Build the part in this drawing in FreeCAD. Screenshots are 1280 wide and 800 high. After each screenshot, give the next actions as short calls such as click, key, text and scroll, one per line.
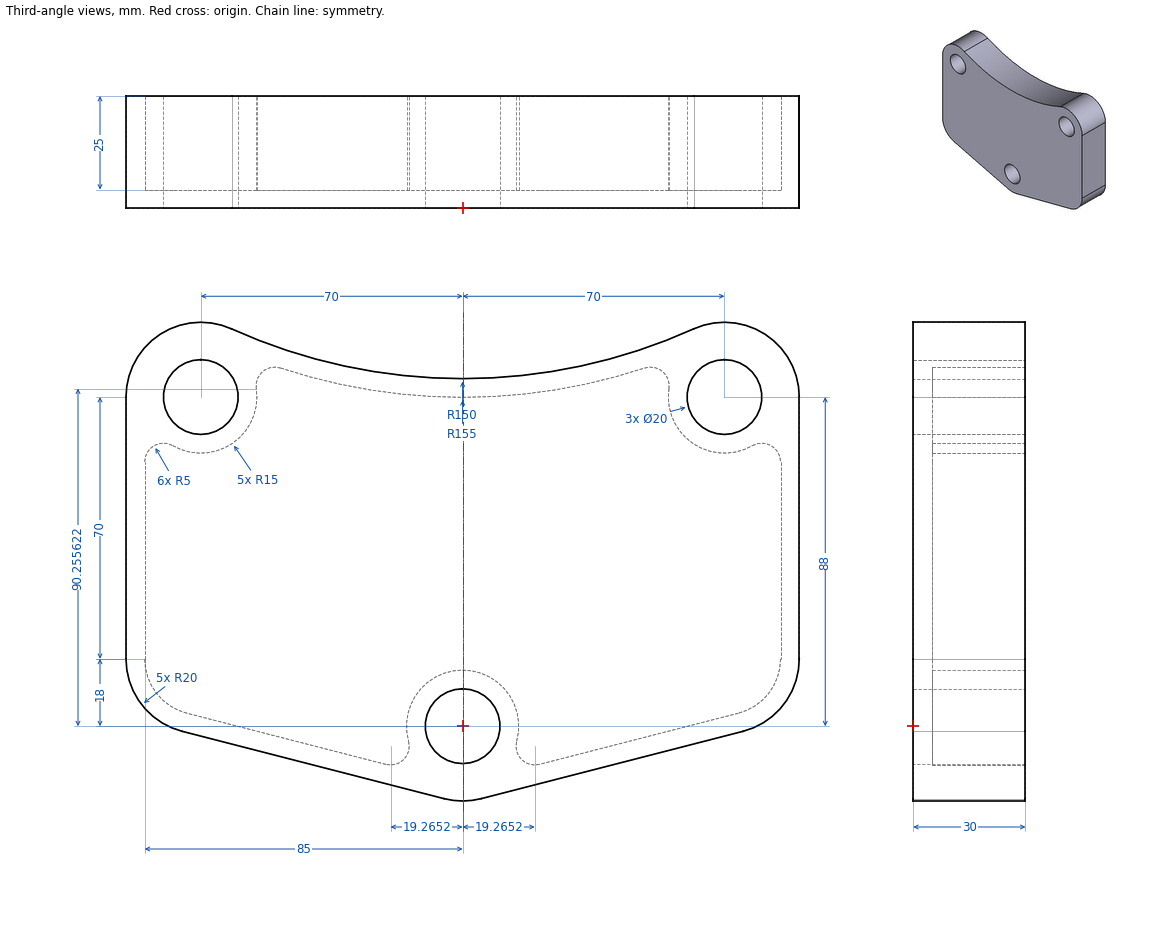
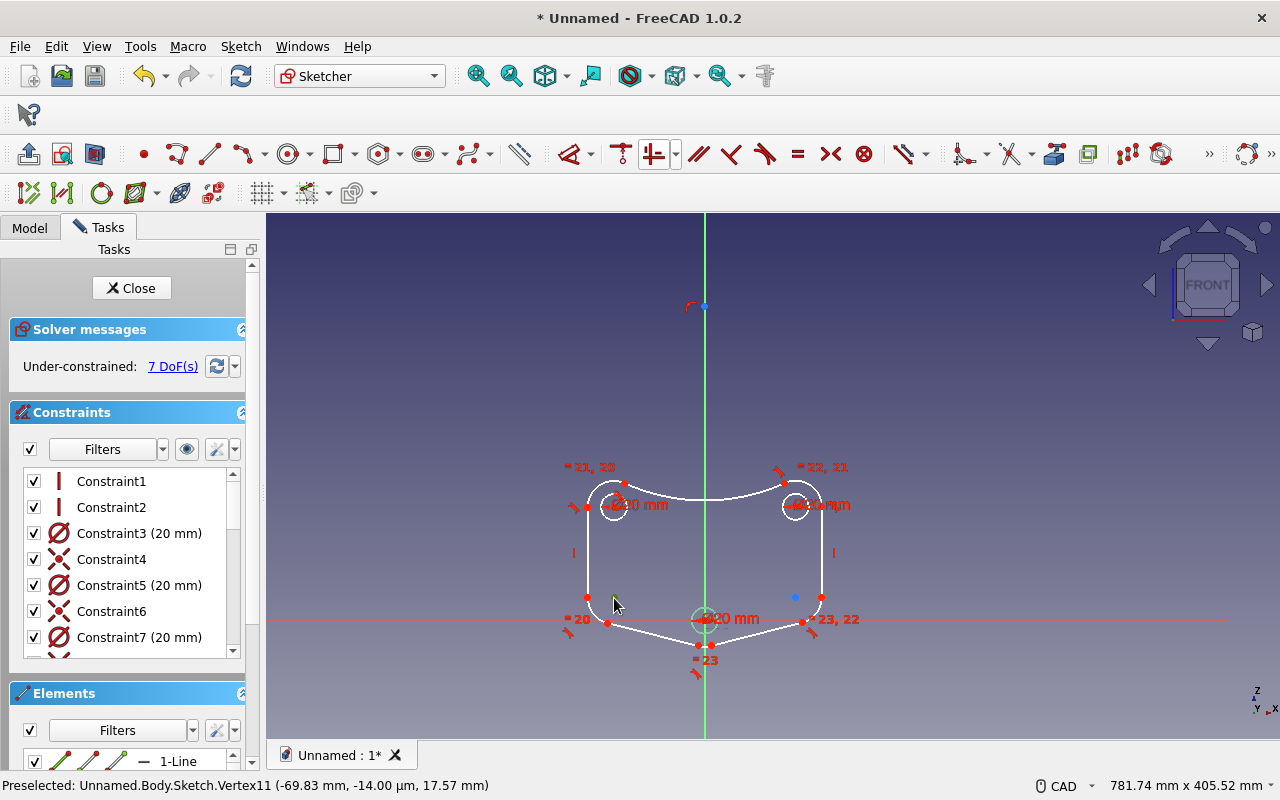
click(796, 597)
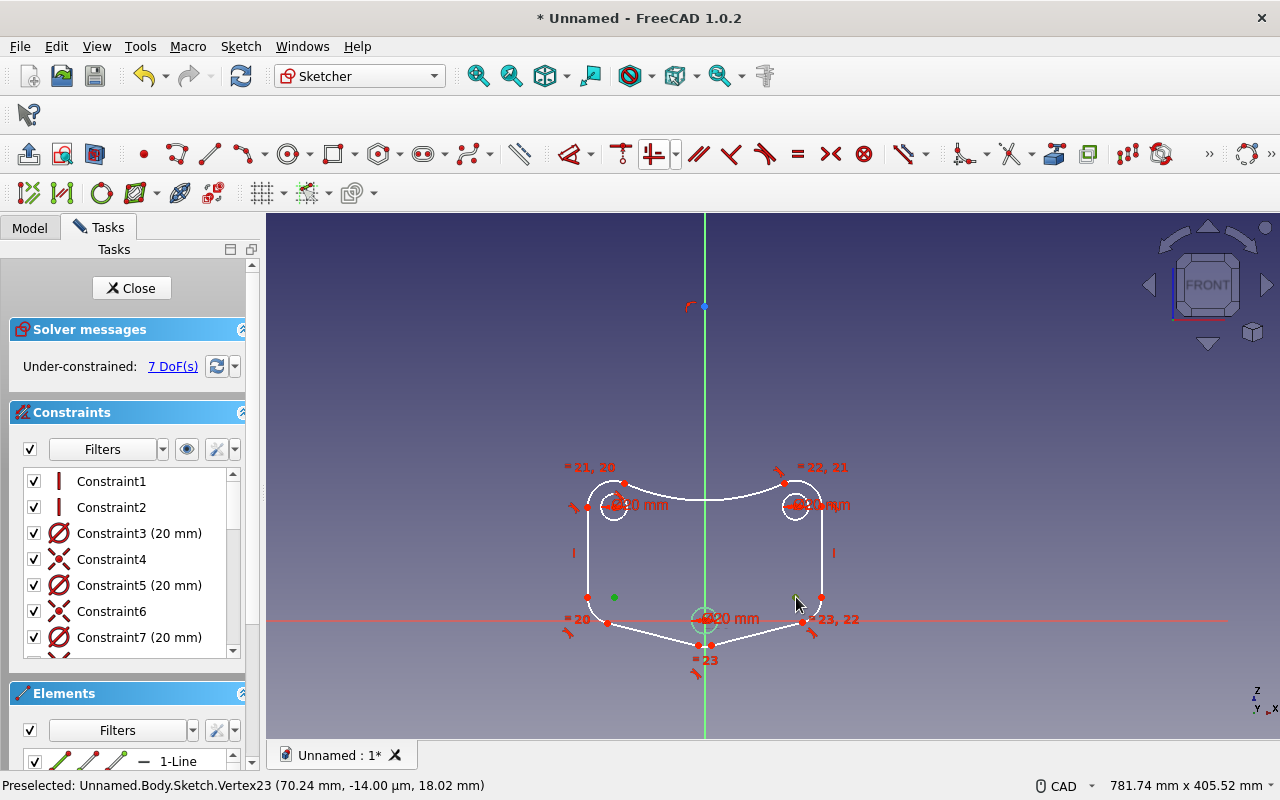
click(705, 577)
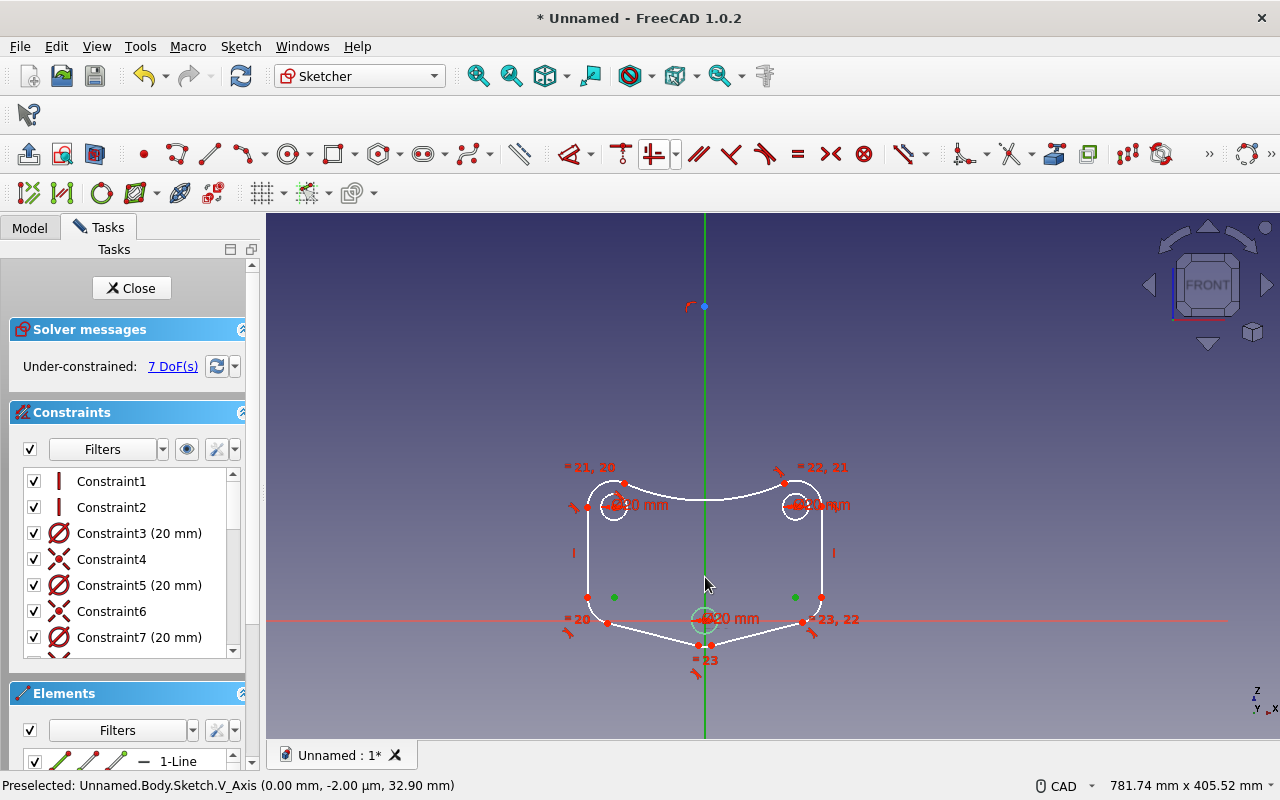
click(831, 154)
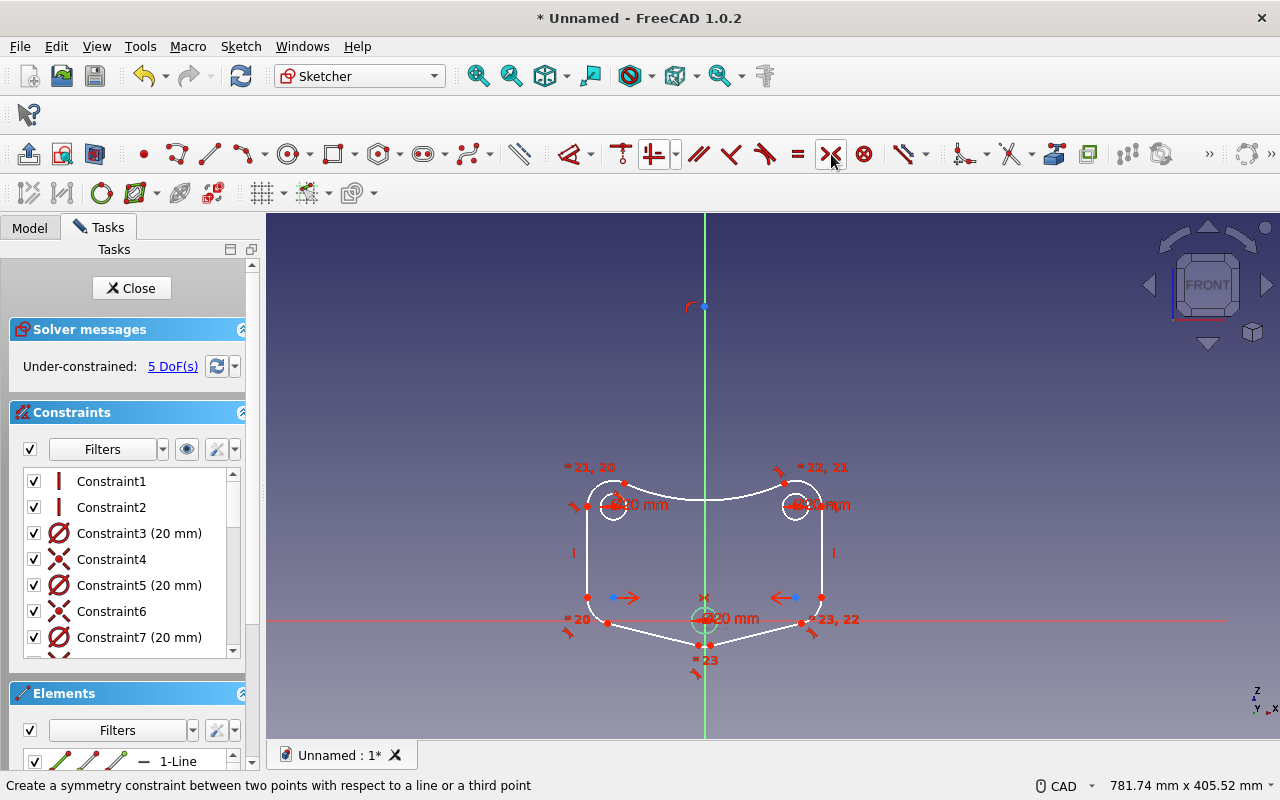
click(568, 154)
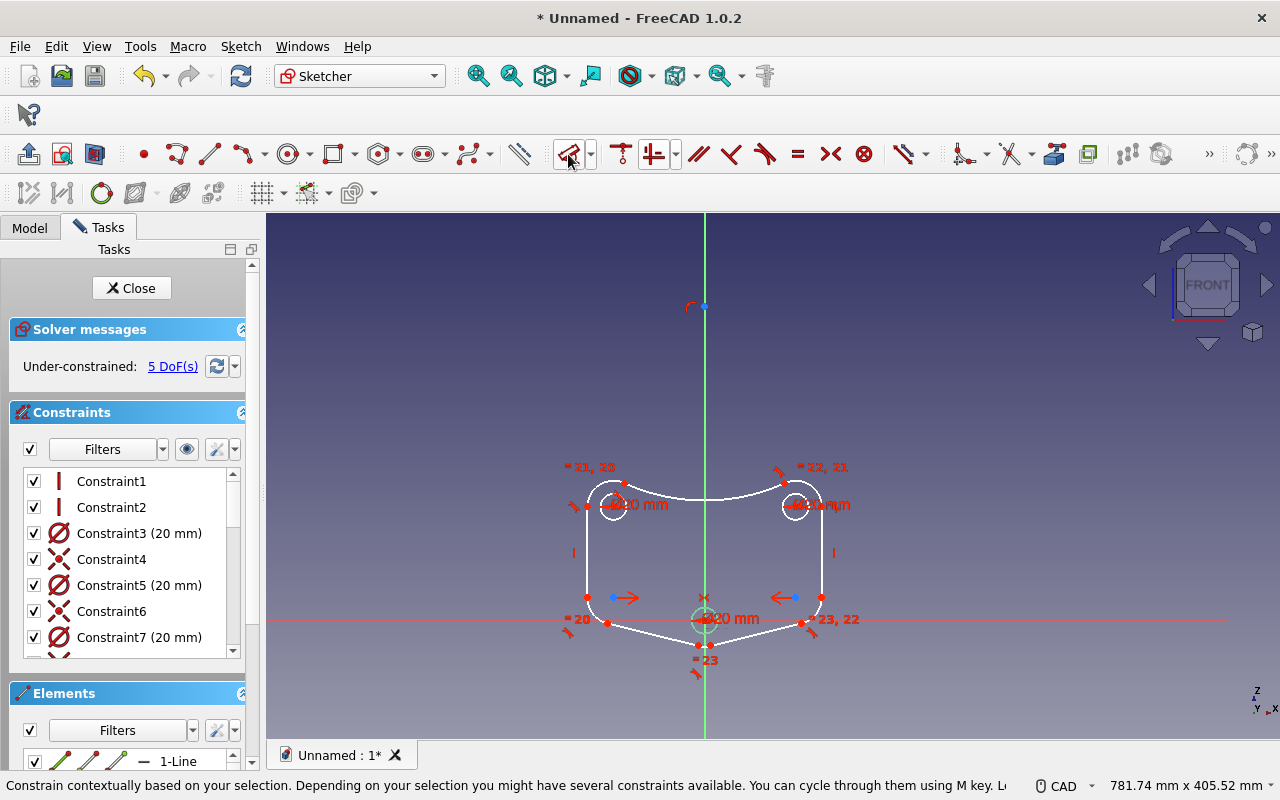
scroll(589, 608, up, 3)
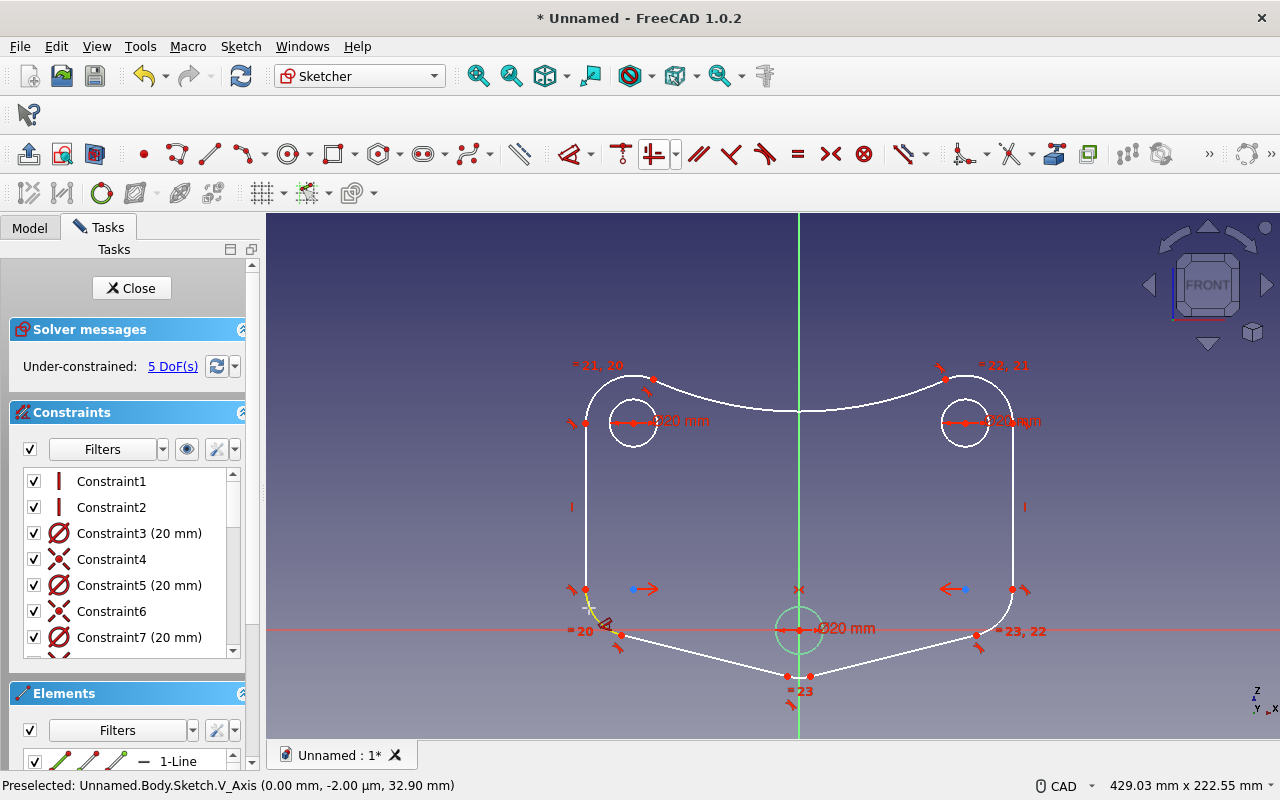
click(590, 607)
click(555, 581)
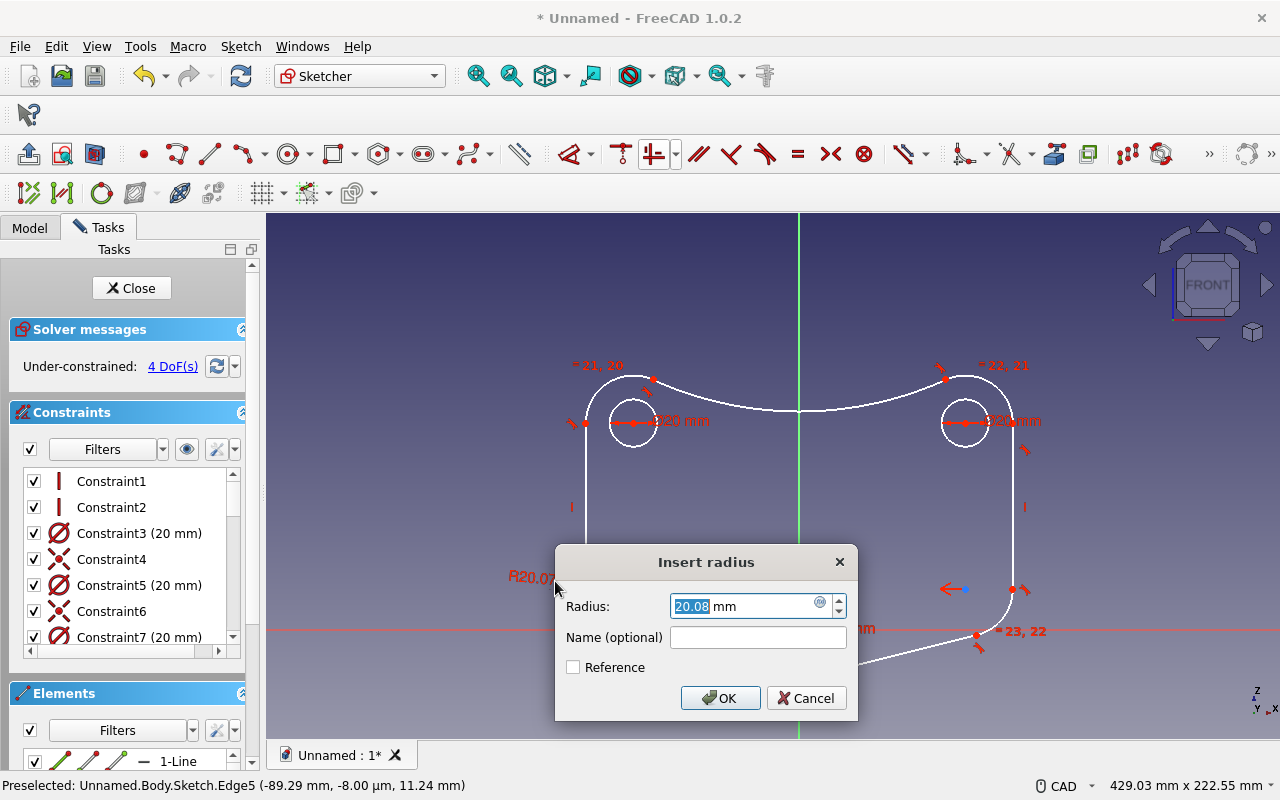
text(20)
key(Return)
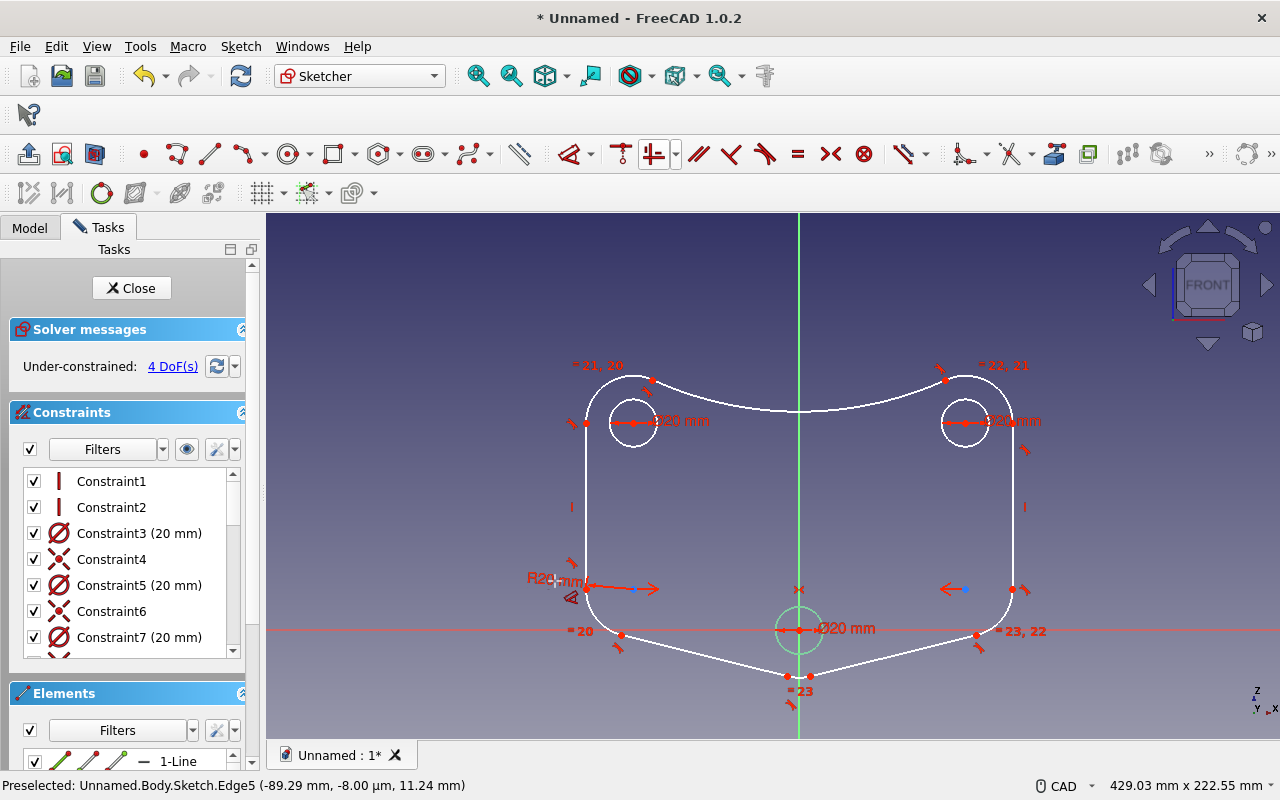
click(739, 407)
click(734, 439)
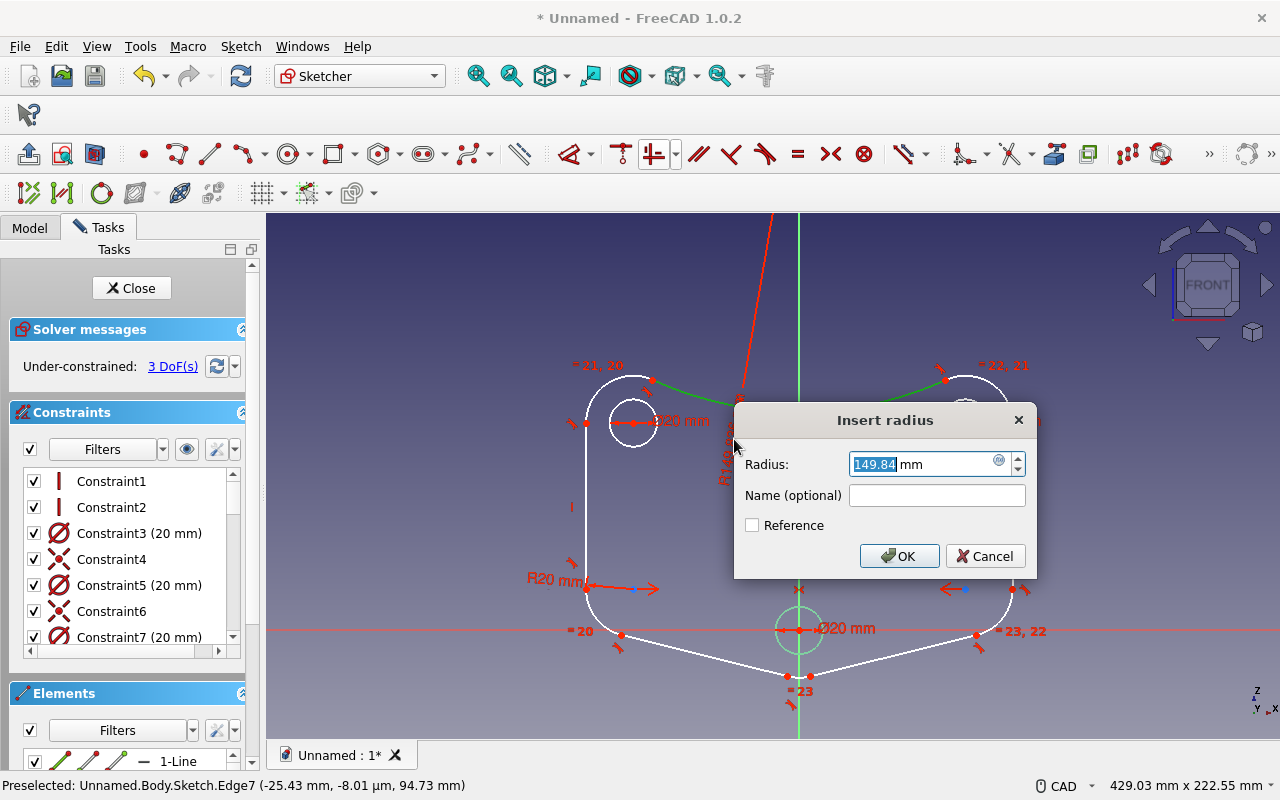
text(150)
key(Return)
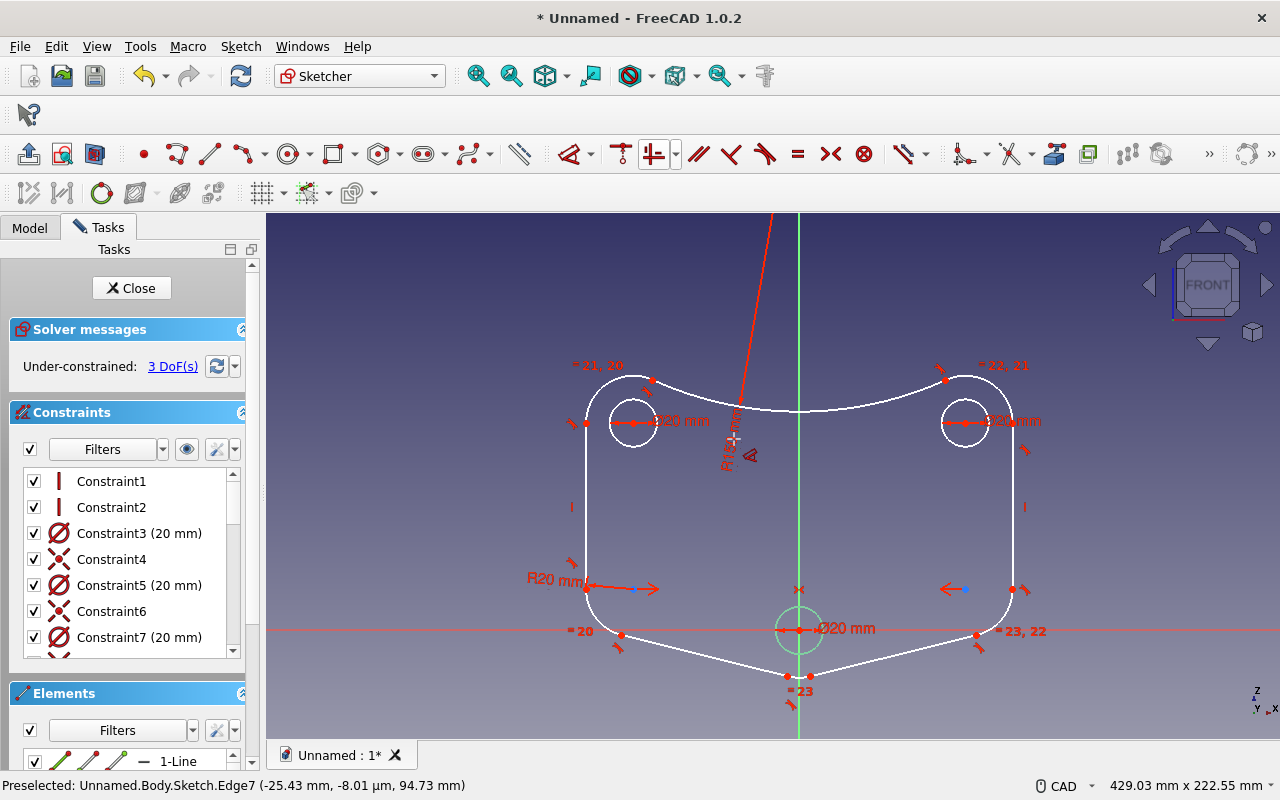
click(586, 539)
click(552, 506)